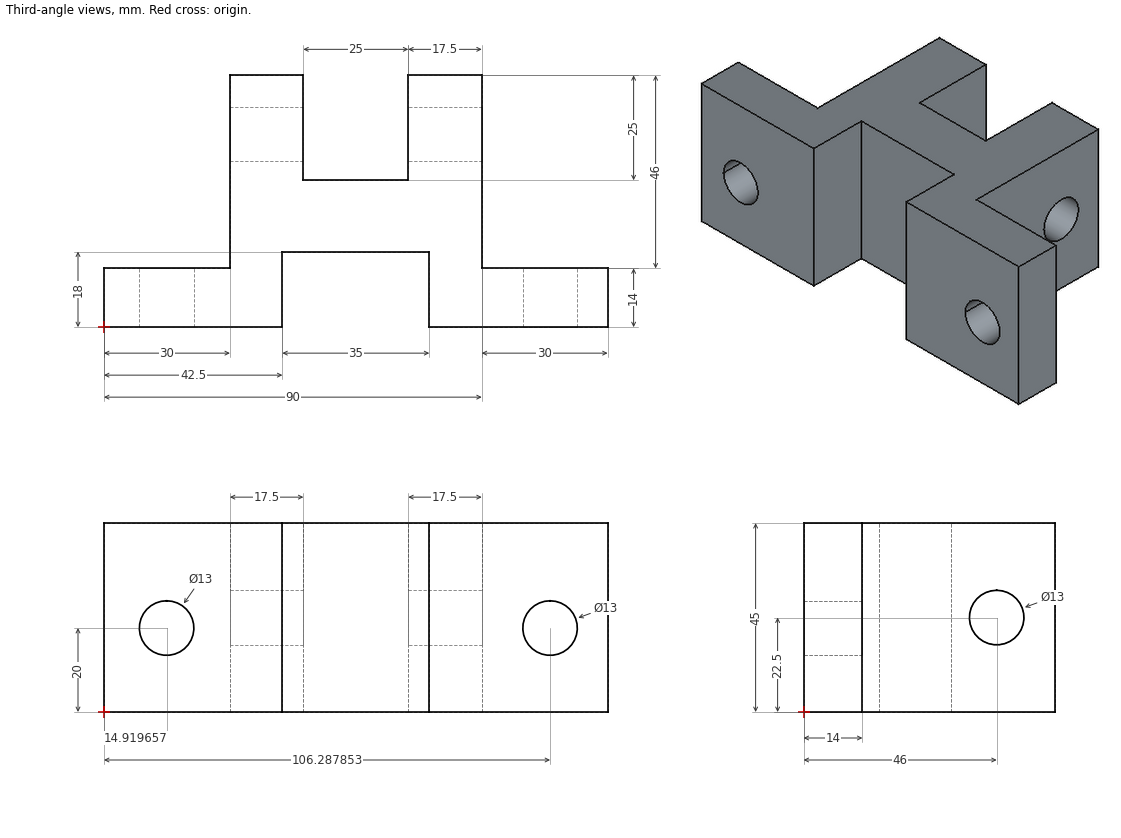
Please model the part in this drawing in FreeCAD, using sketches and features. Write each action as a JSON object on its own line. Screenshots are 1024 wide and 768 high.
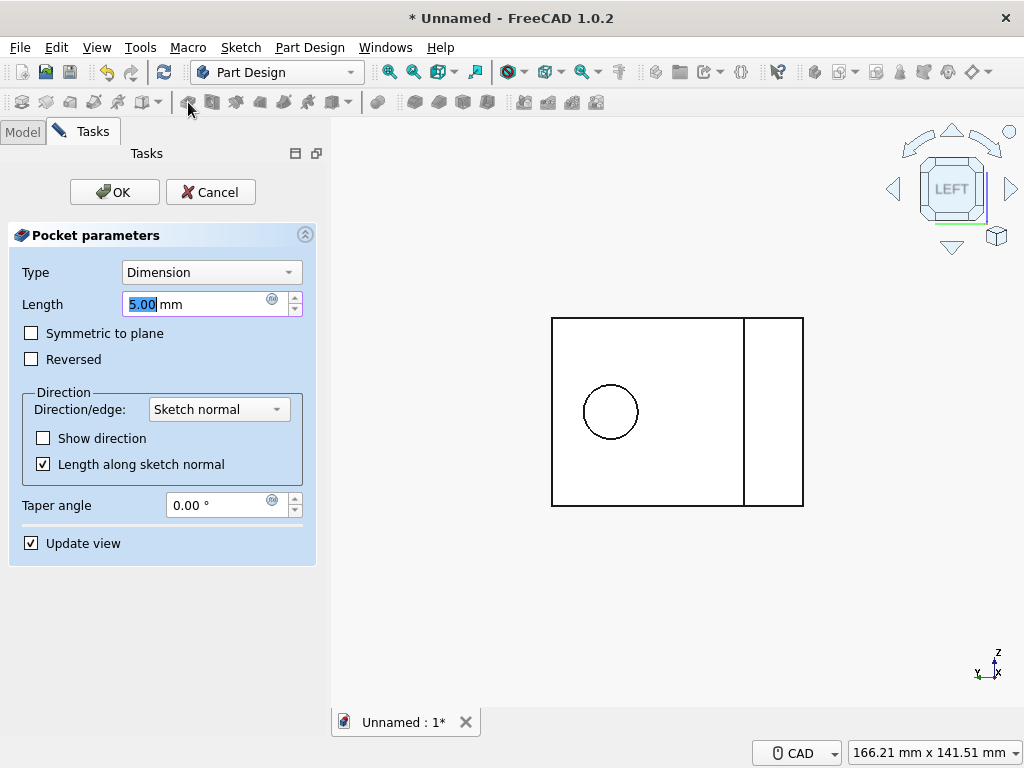
{"action": "type", "text": "17.5"}
{"action": "key", "text": "Tab"}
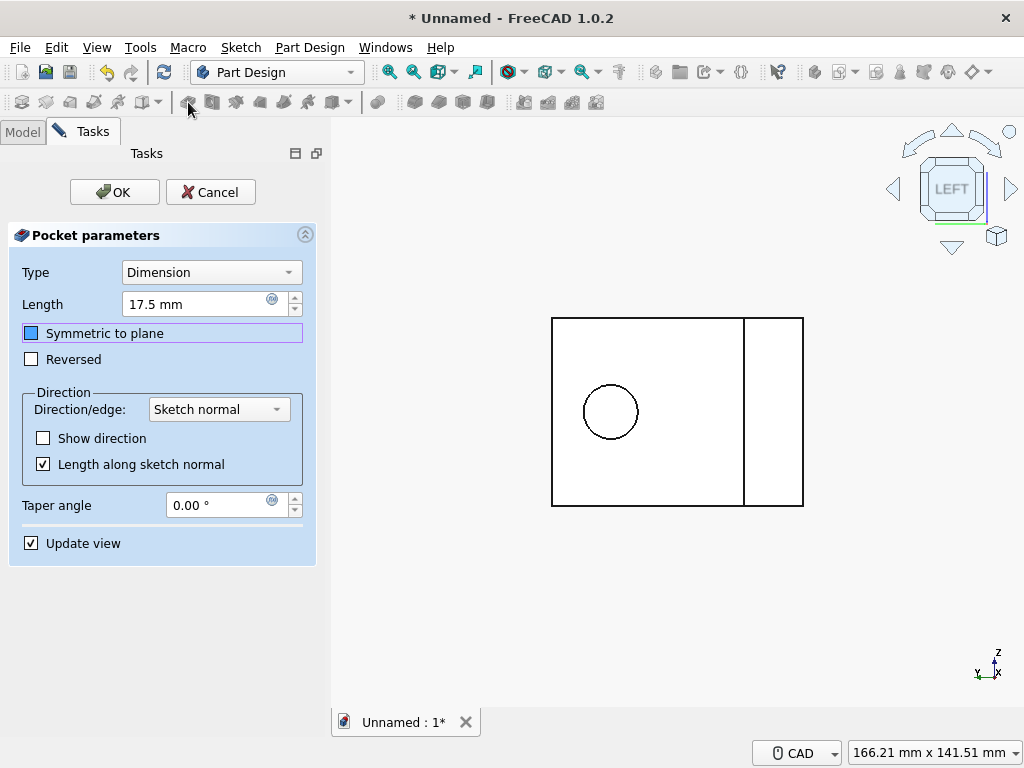
{"action": "left_click", "coordinate": [115, 192]}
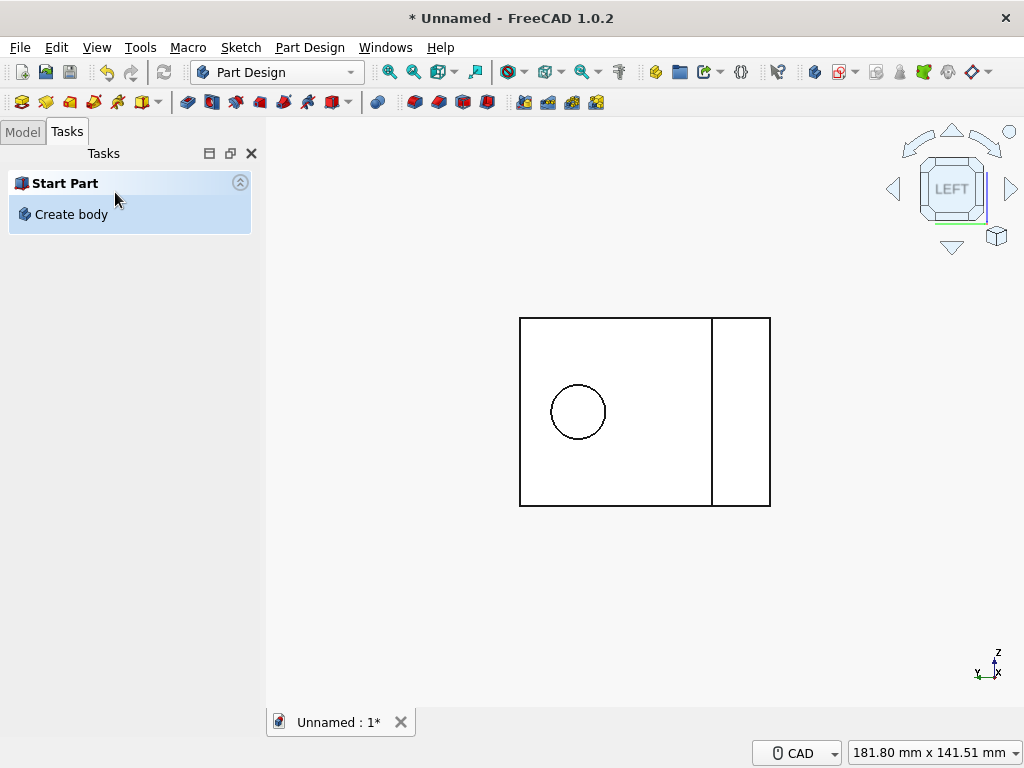
{"action": "left_click", "coordinate": [390, 72]}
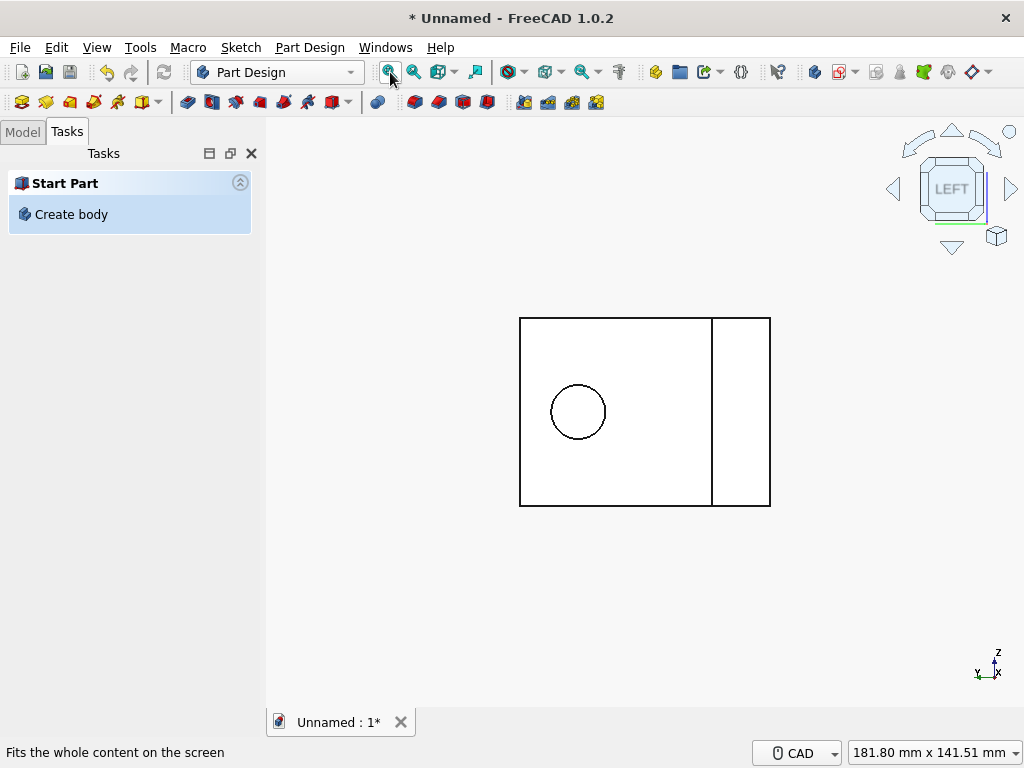
{"action": "left_click", "coordinate": [572, 411]}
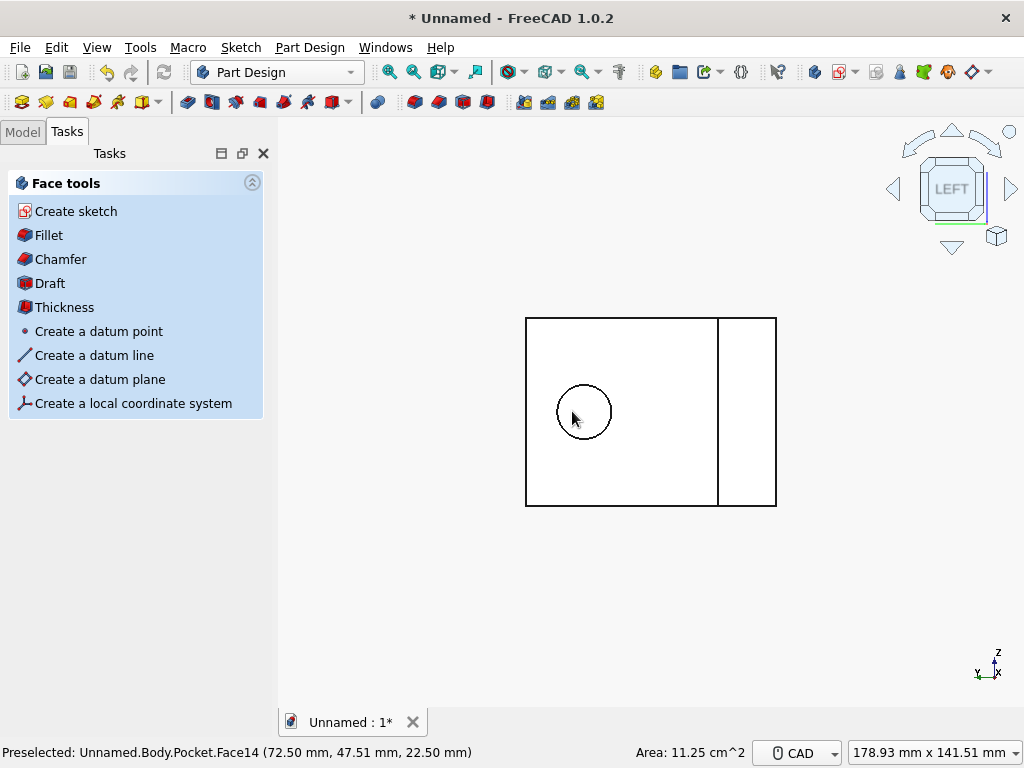
{"action": "left_click", "coordinate": [840, 72]}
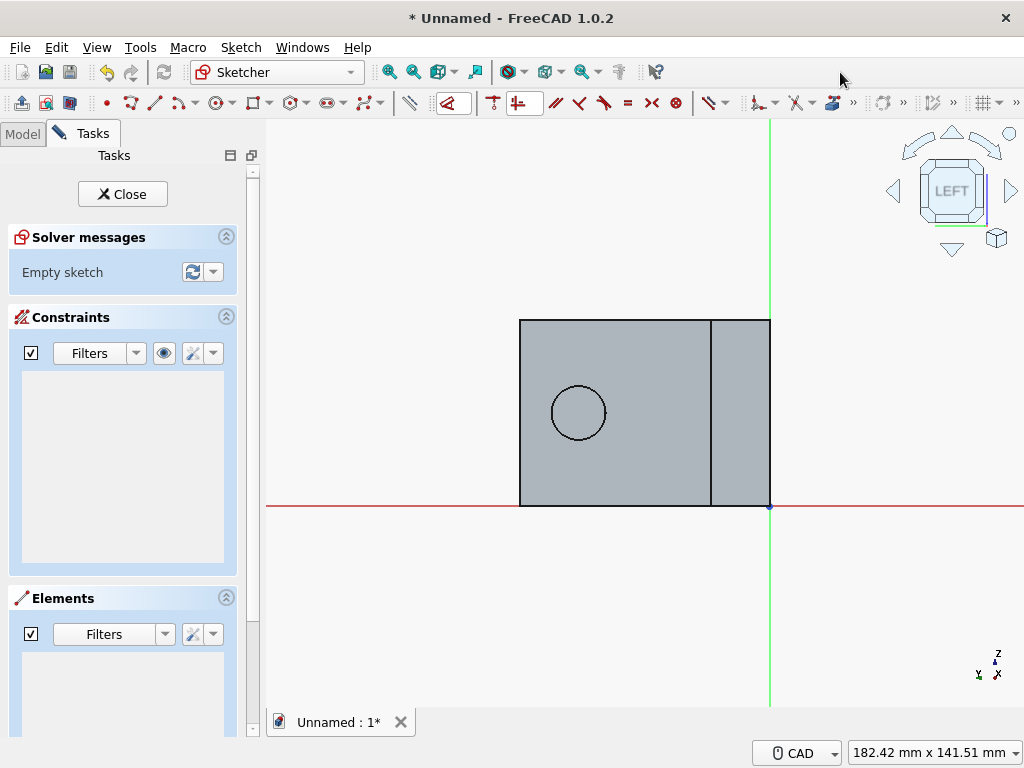
{"action": "left_click", "coordinate": [70, 104]}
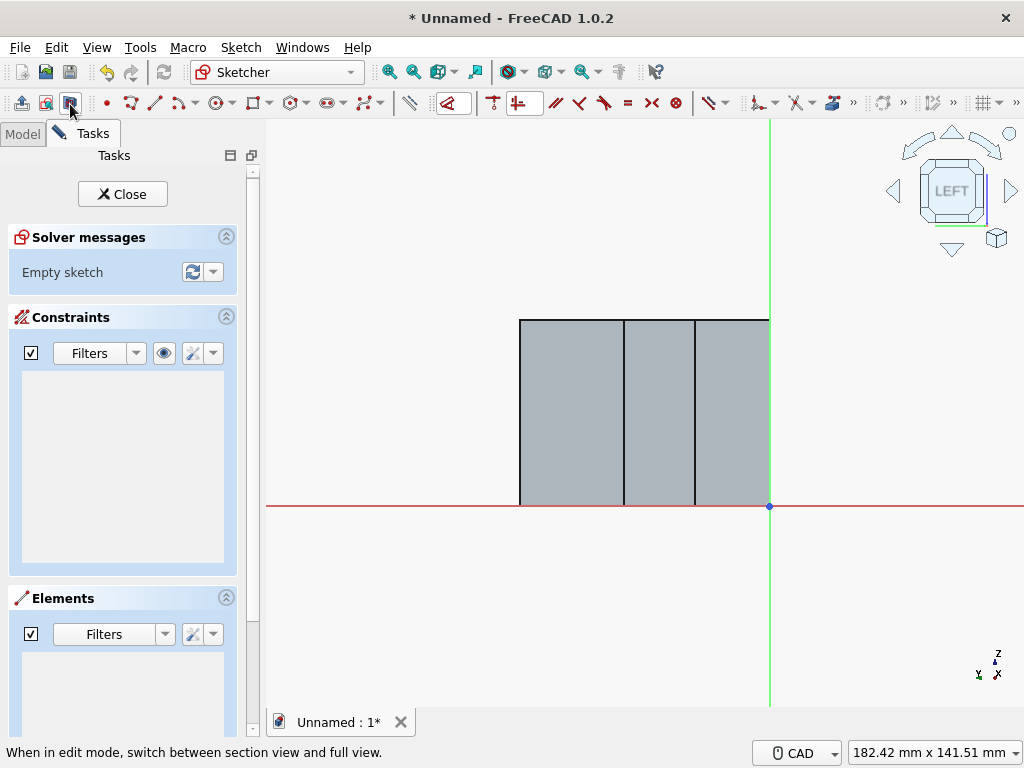
{"action": "scroll", "coordinate": [579, 413], "scroll_direction": "up", "scroll_amount": 10}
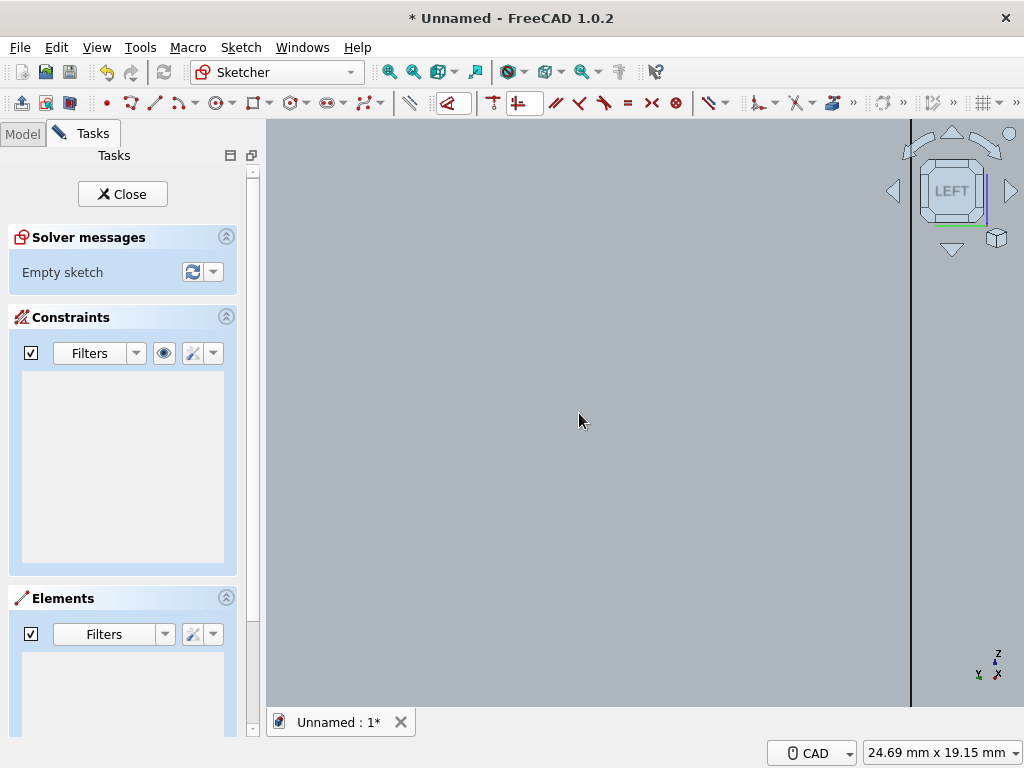
{"action": "left_click", "coordinate": [216, 104]}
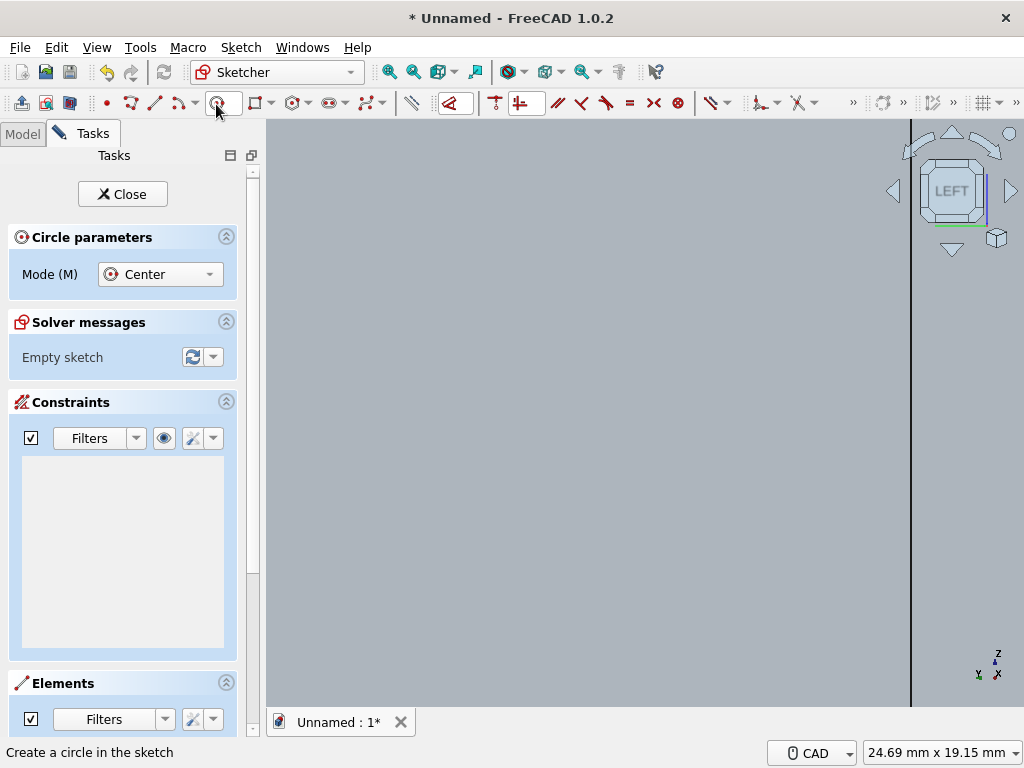
{"action": "left_click", "coordinate": [573, 410]}
{"action": "mouse_move", "coordinate": [714, 269]}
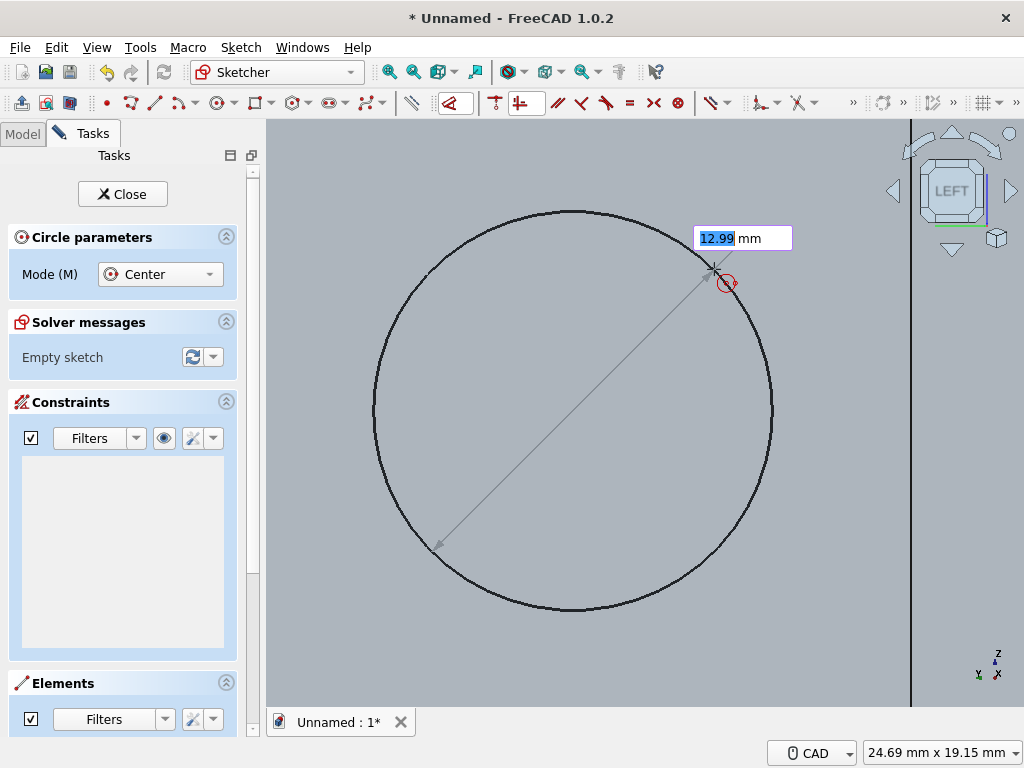
{"action": "type", "text": "13"}
{"action": "key", "text": "Return"}
{"action": "key", "text": "Escape"}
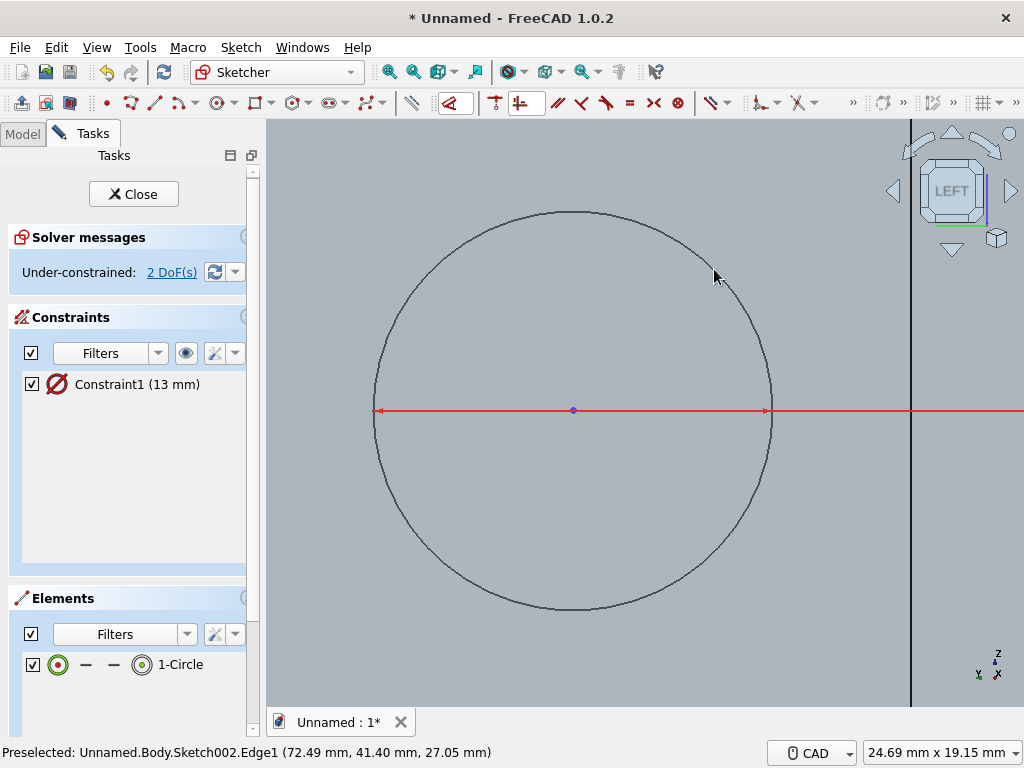
{"action": "left_click", "coordinate": [573, 411]}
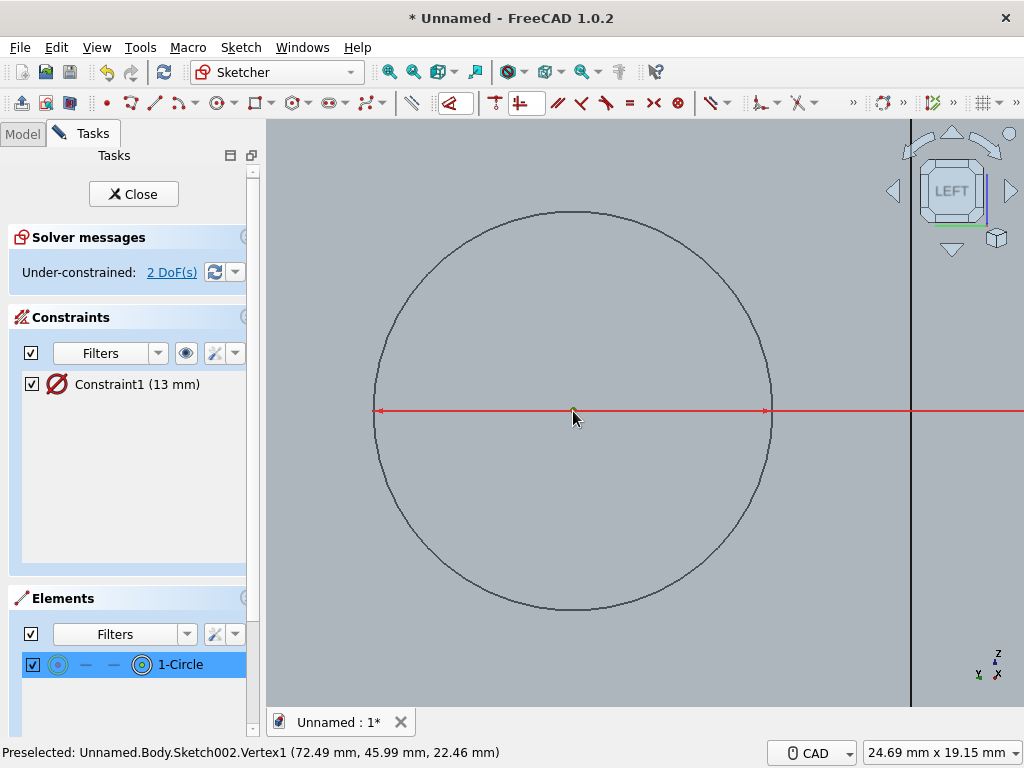
{"action": "key", "text": "l"}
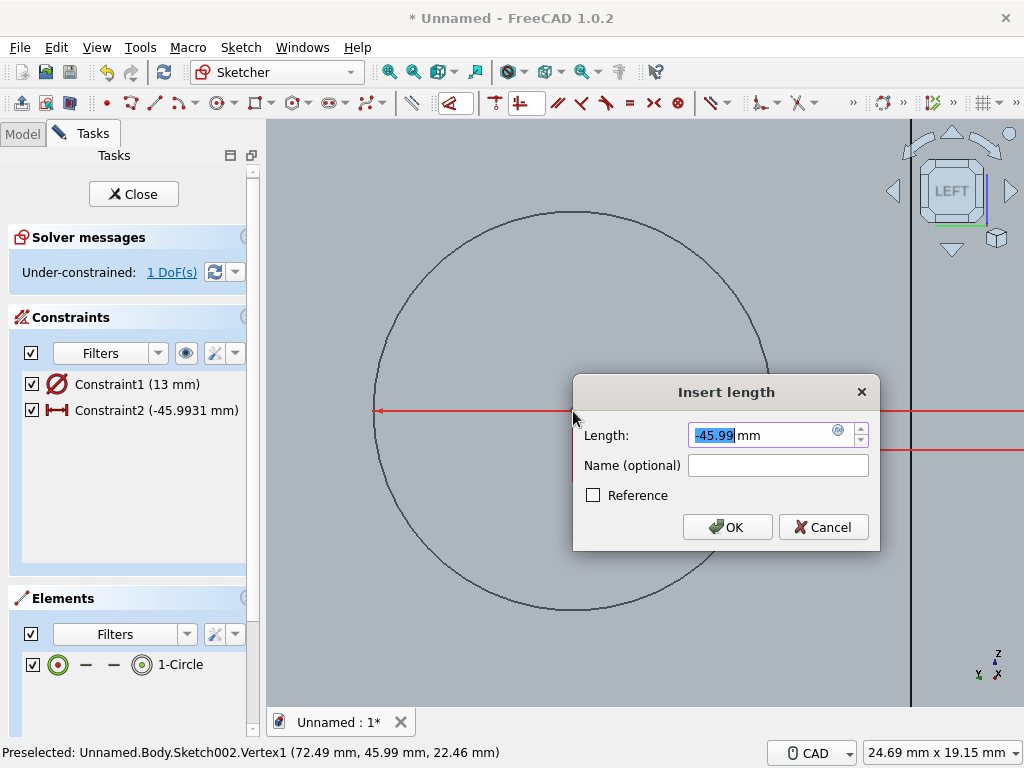
{"action": "type", "text": "-46"}
{"action": "key", "text": "Return"}